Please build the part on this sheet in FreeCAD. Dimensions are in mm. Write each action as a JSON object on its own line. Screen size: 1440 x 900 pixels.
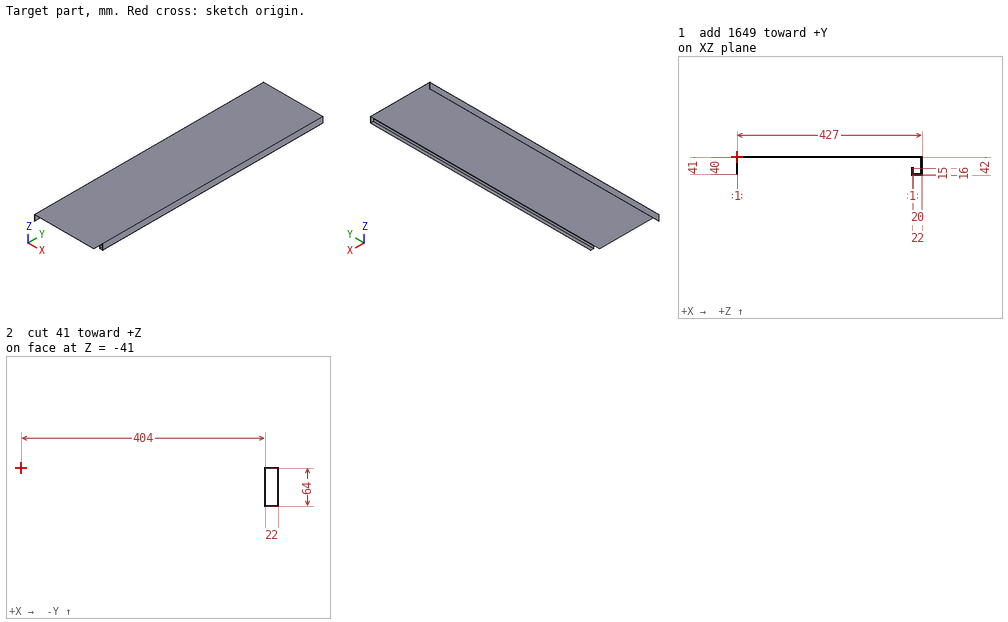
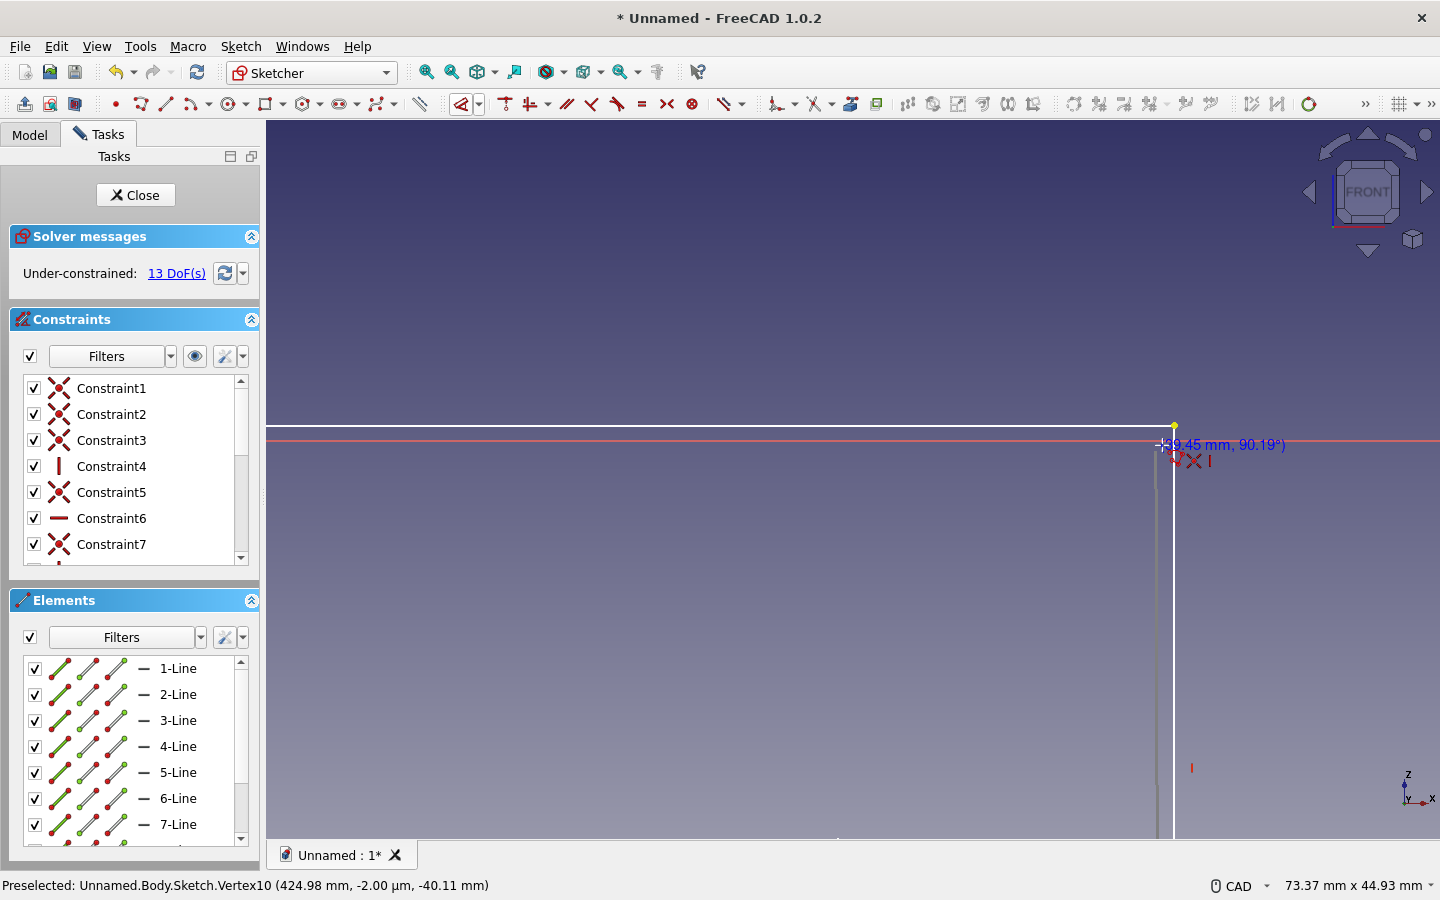
{"action": "left_click", "coordinate": [1158, 450]}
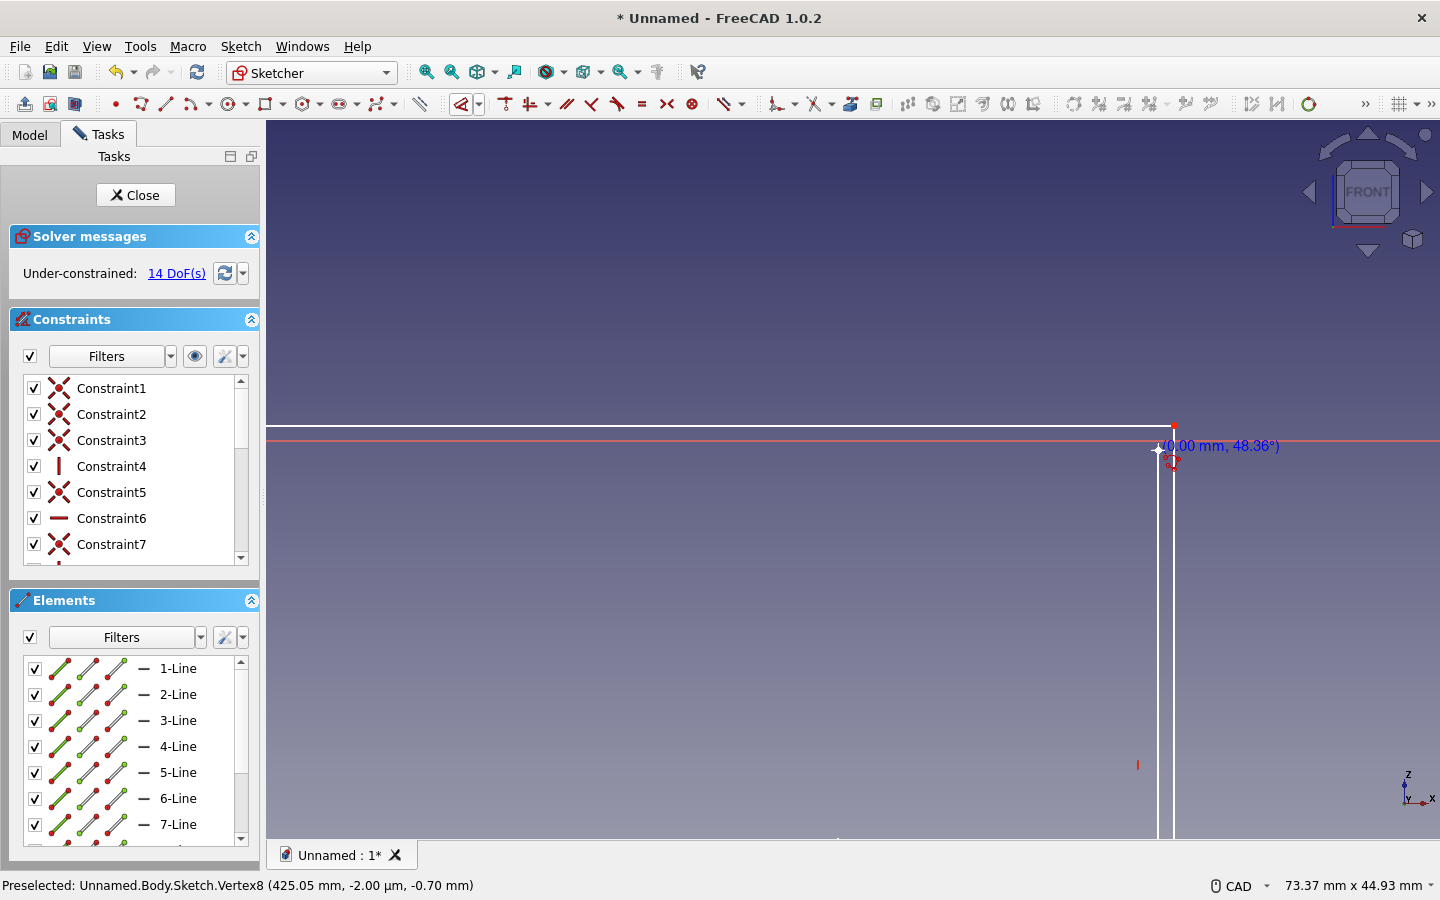
{"action": "scroll", "coordinate": [1162, 444], "scroll_direction": "down", "scroll_amount": 11}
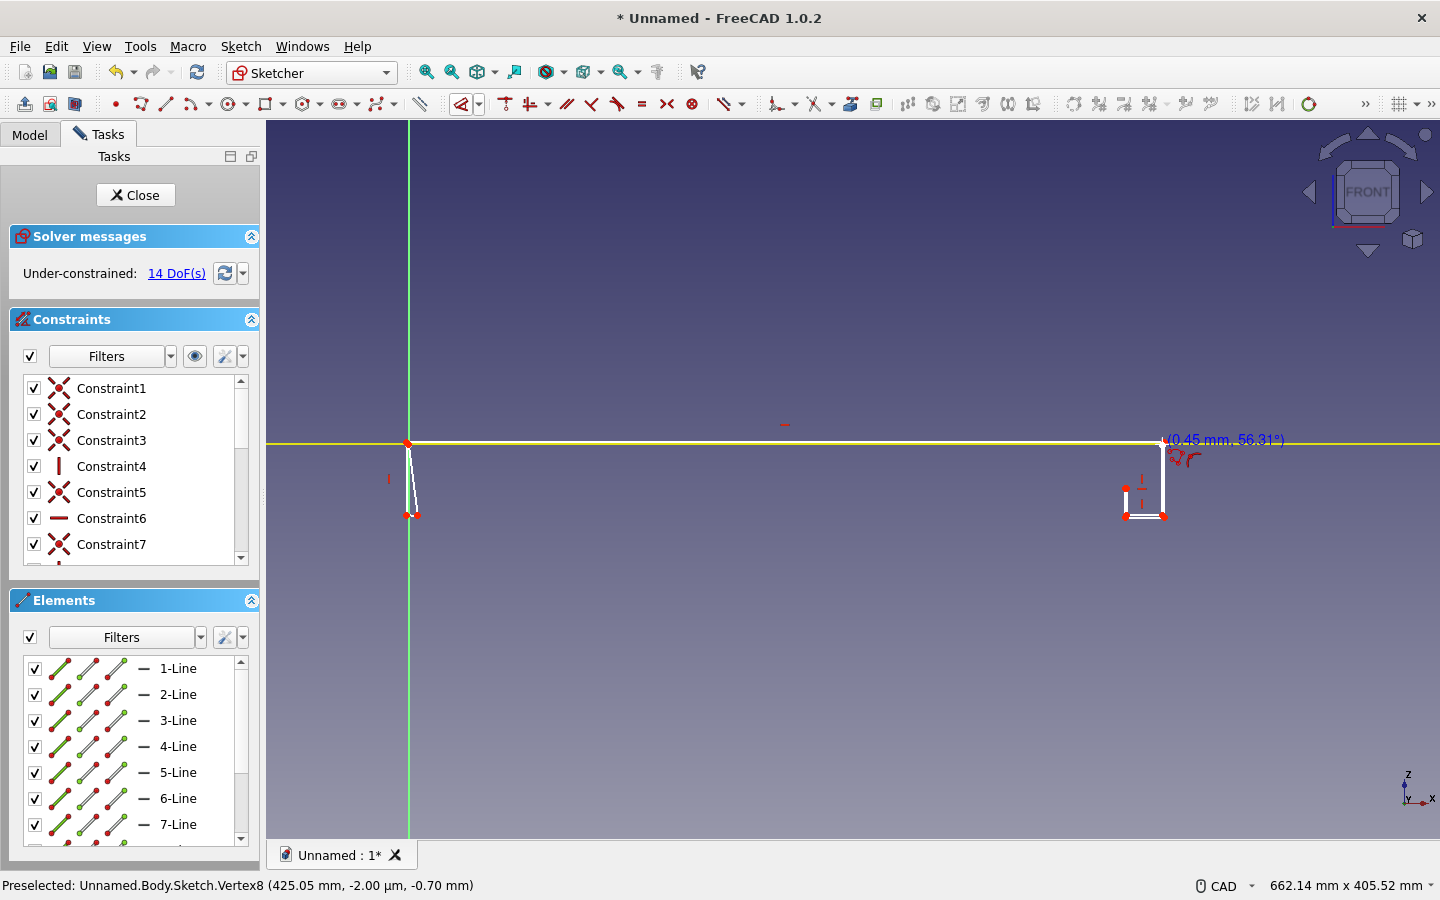
{"action": "scroll", "coordinate": [409, 444], "scroll_direction": "up", "scroll_amount": 11}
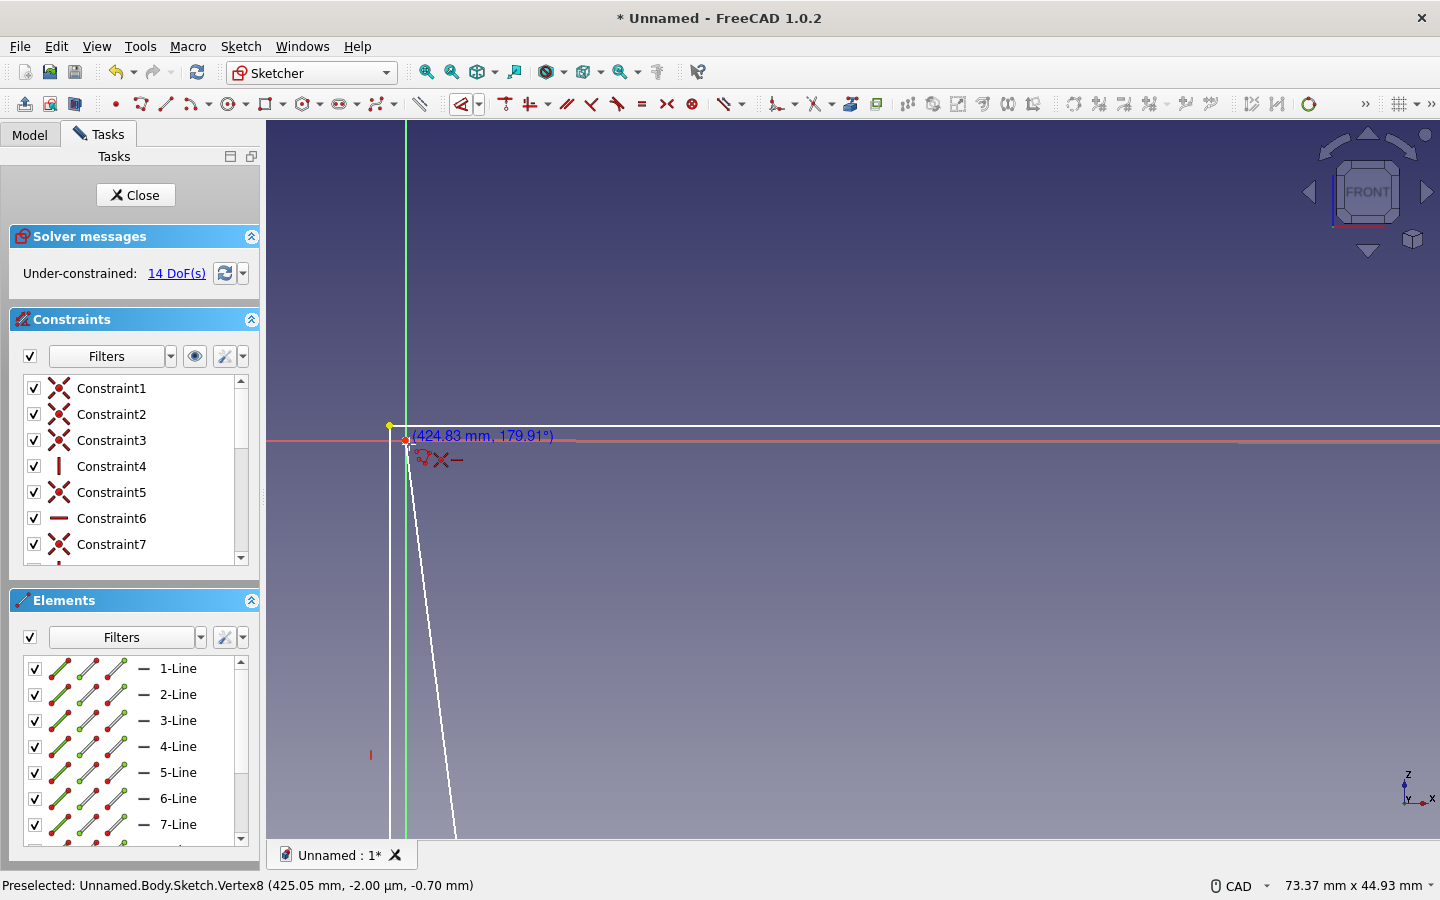
{"action": "left_click", "coordinate": [406, 441]}
{"action": "key", "text": "Escape"}
{"action": "key", "text": "Escape"}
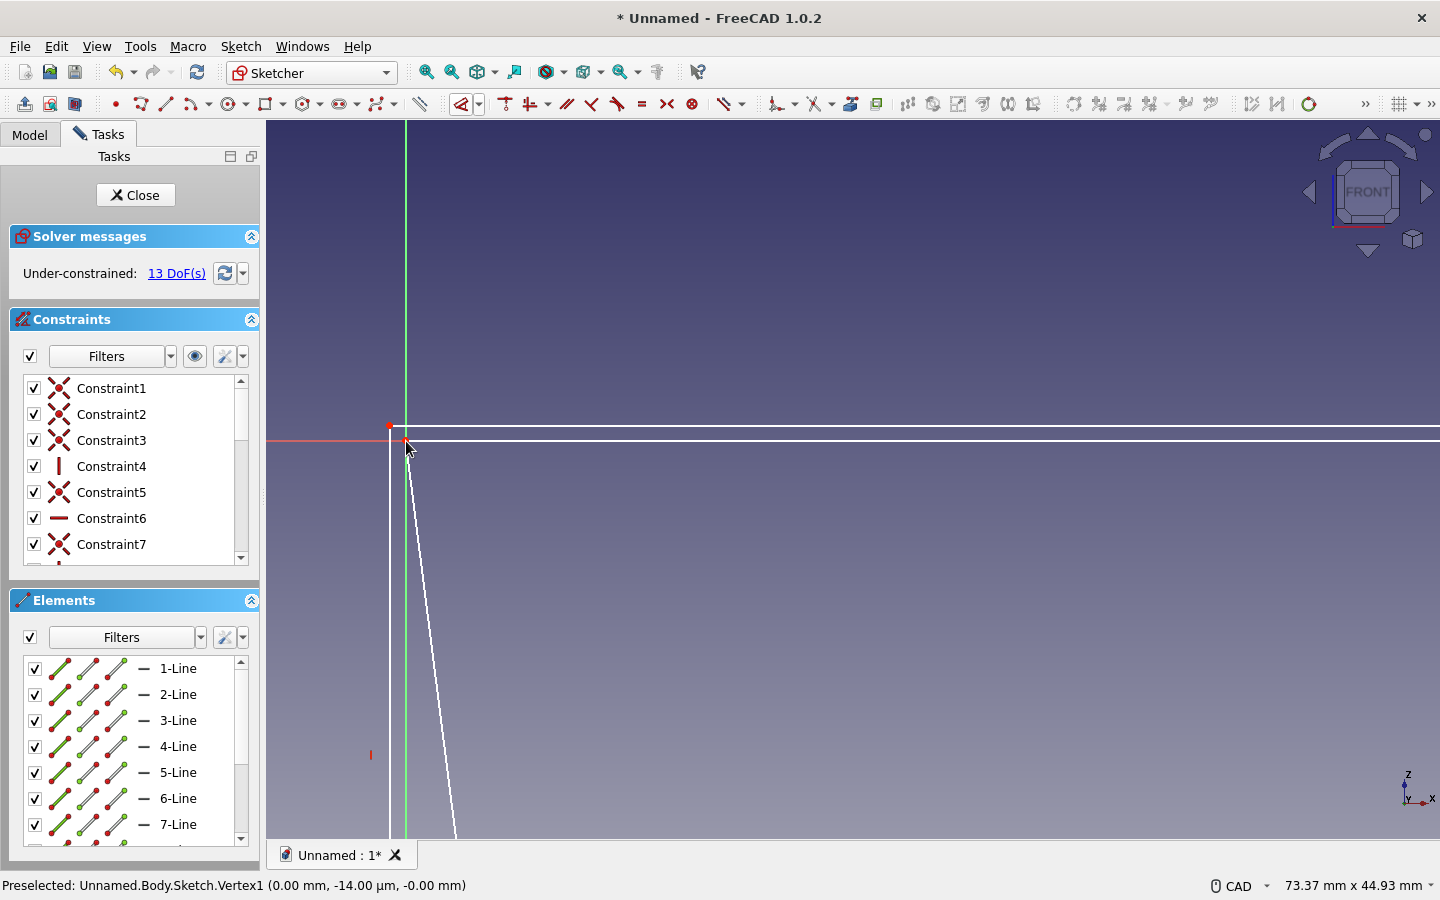
{"action": "left_click", "coordinate": [430, 636]}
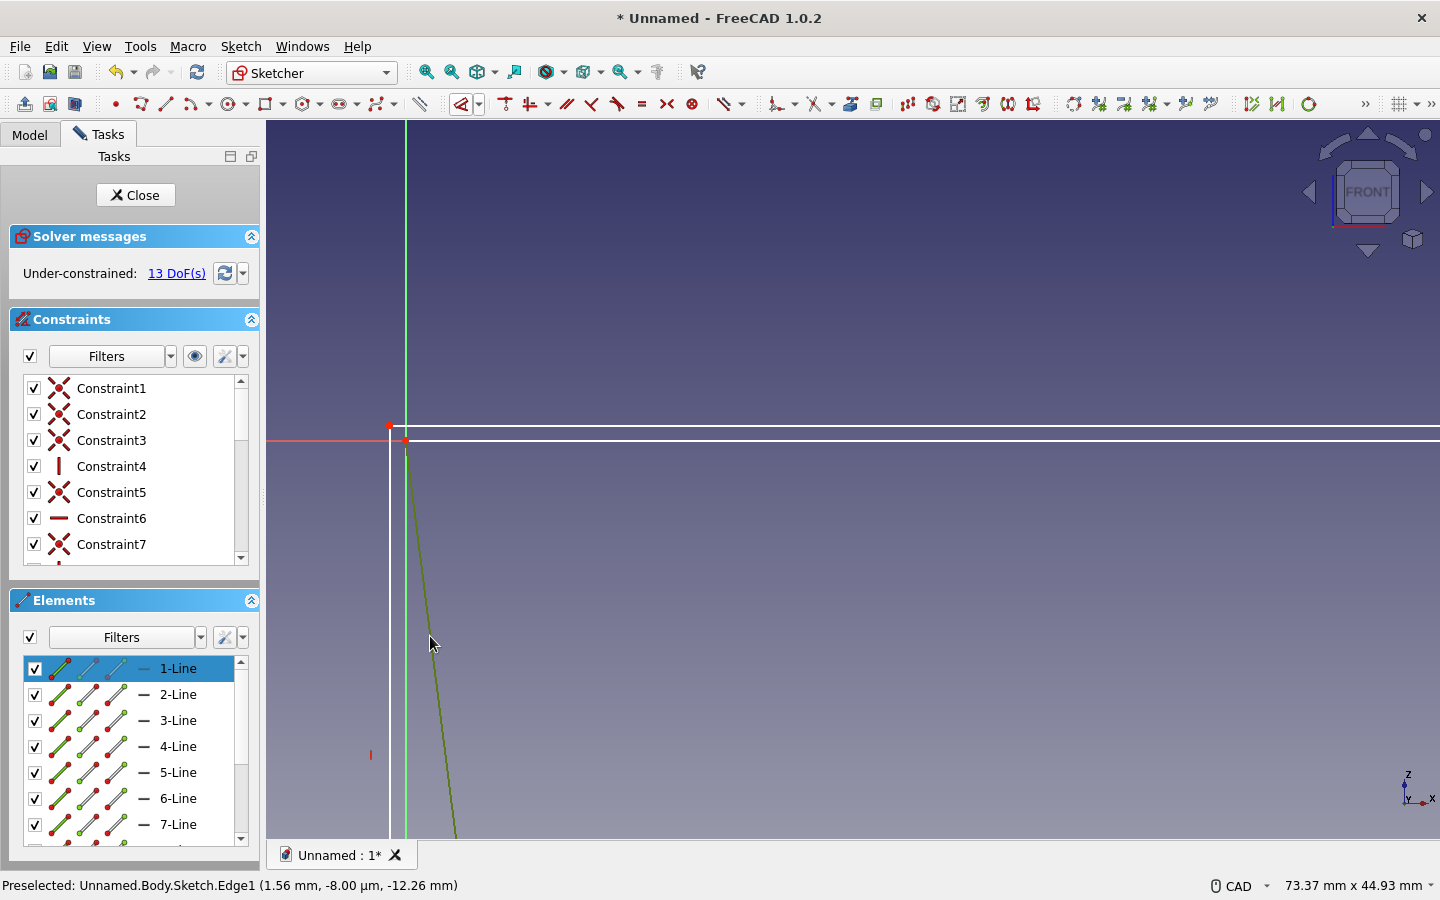
{"action": "key", "text": "v"}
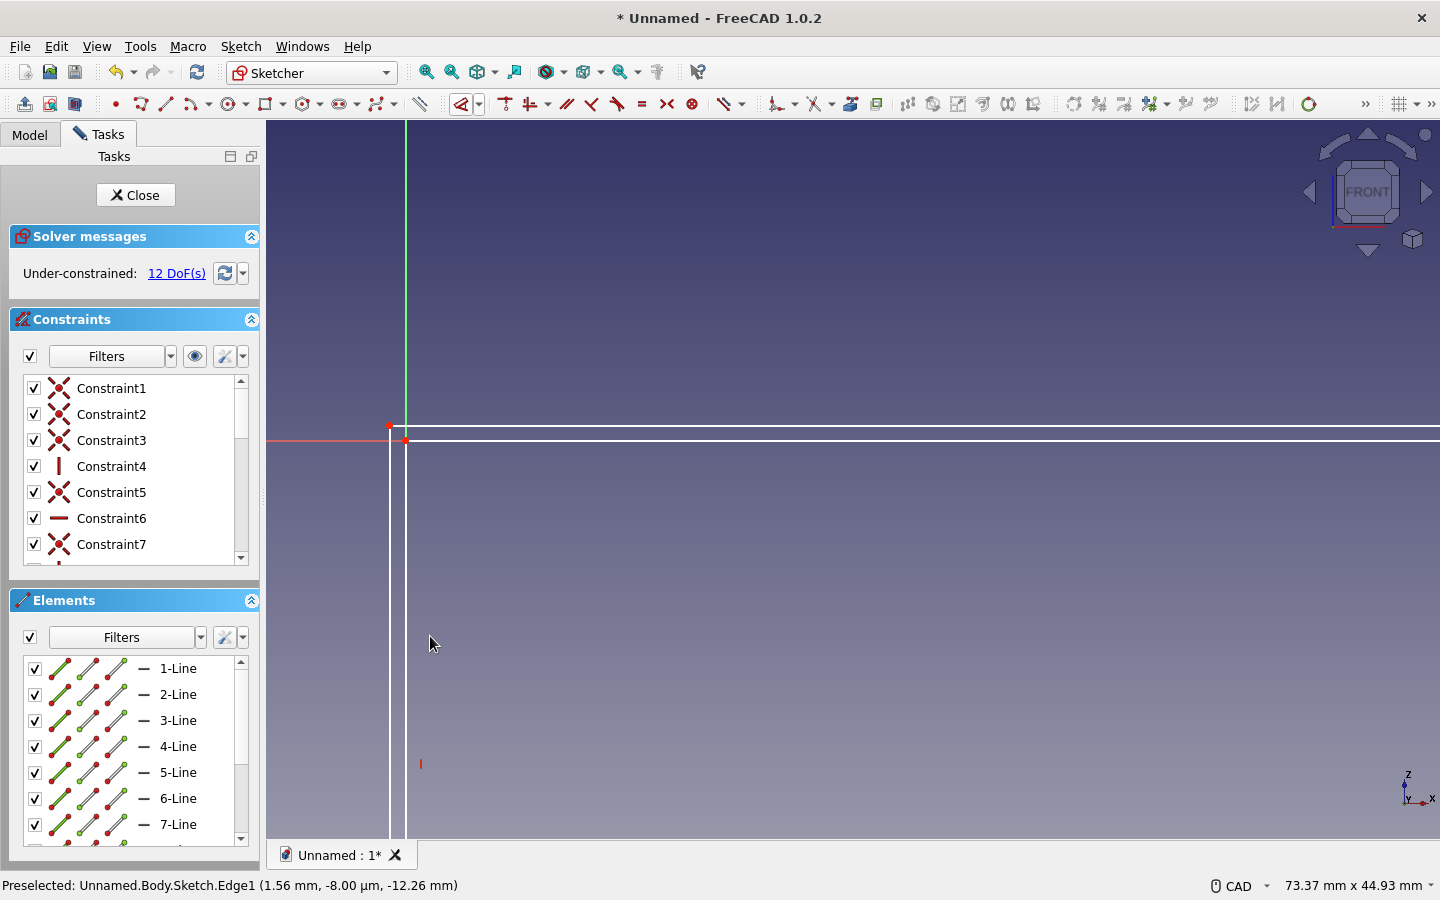
{"action": "scroll", "coordinate": [408, 444], "scroll_direction": "down", "scroll_amount": 11}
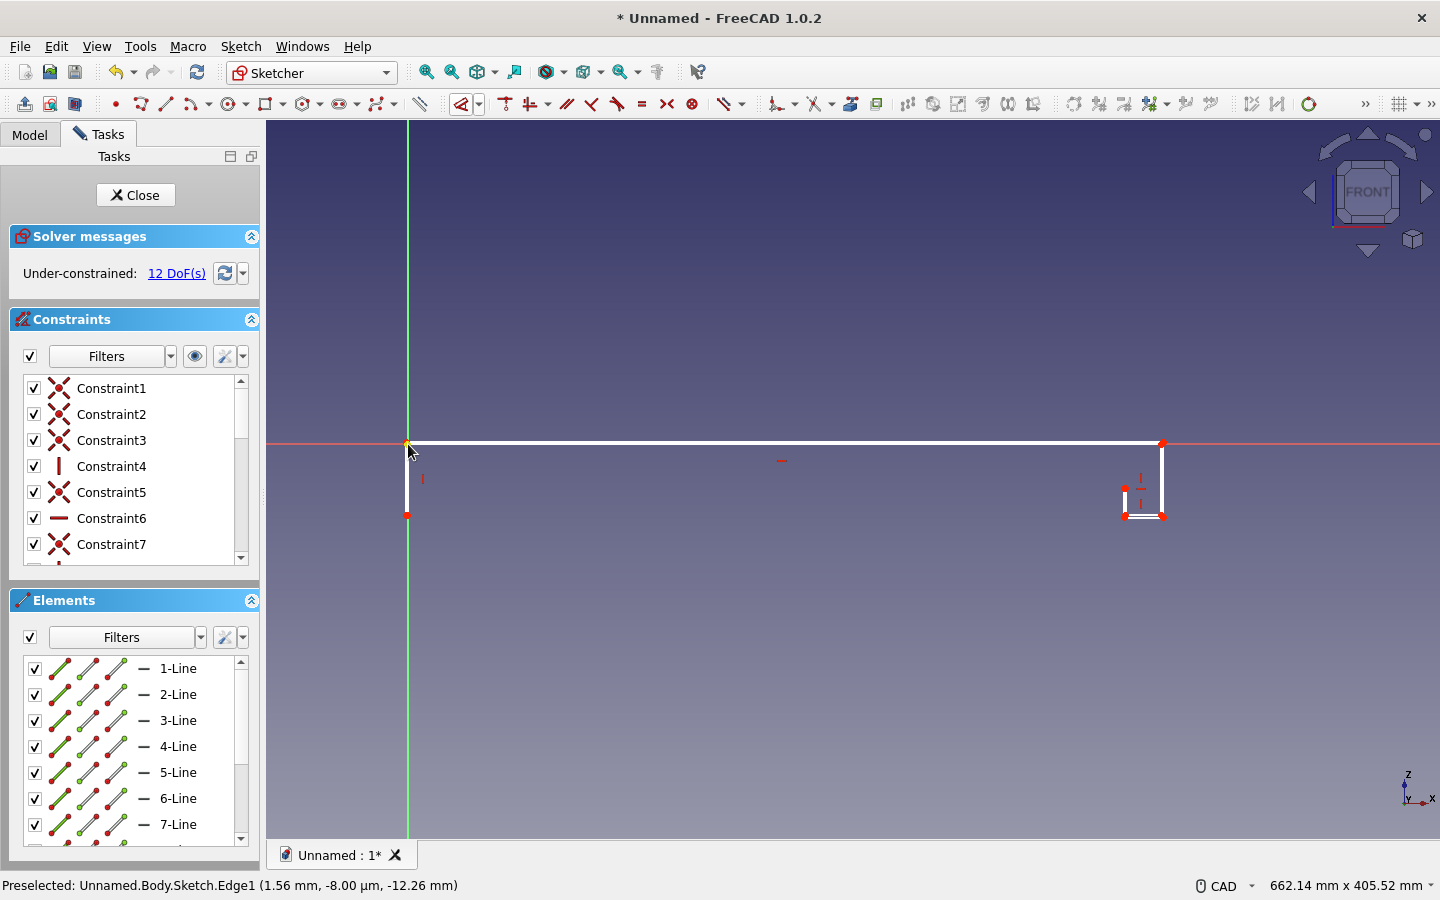
{"action": "scroll", "coordinate": [407, 516], "scroll_direction": "up", "scroll_amount": 14}